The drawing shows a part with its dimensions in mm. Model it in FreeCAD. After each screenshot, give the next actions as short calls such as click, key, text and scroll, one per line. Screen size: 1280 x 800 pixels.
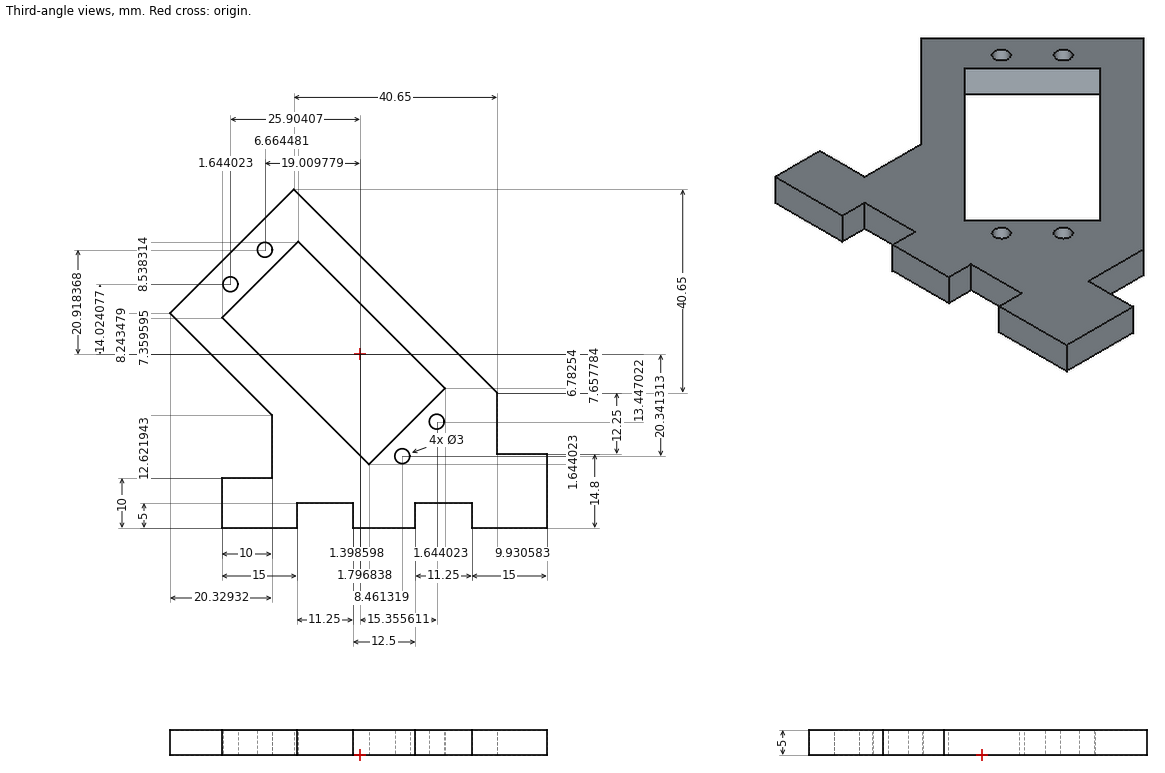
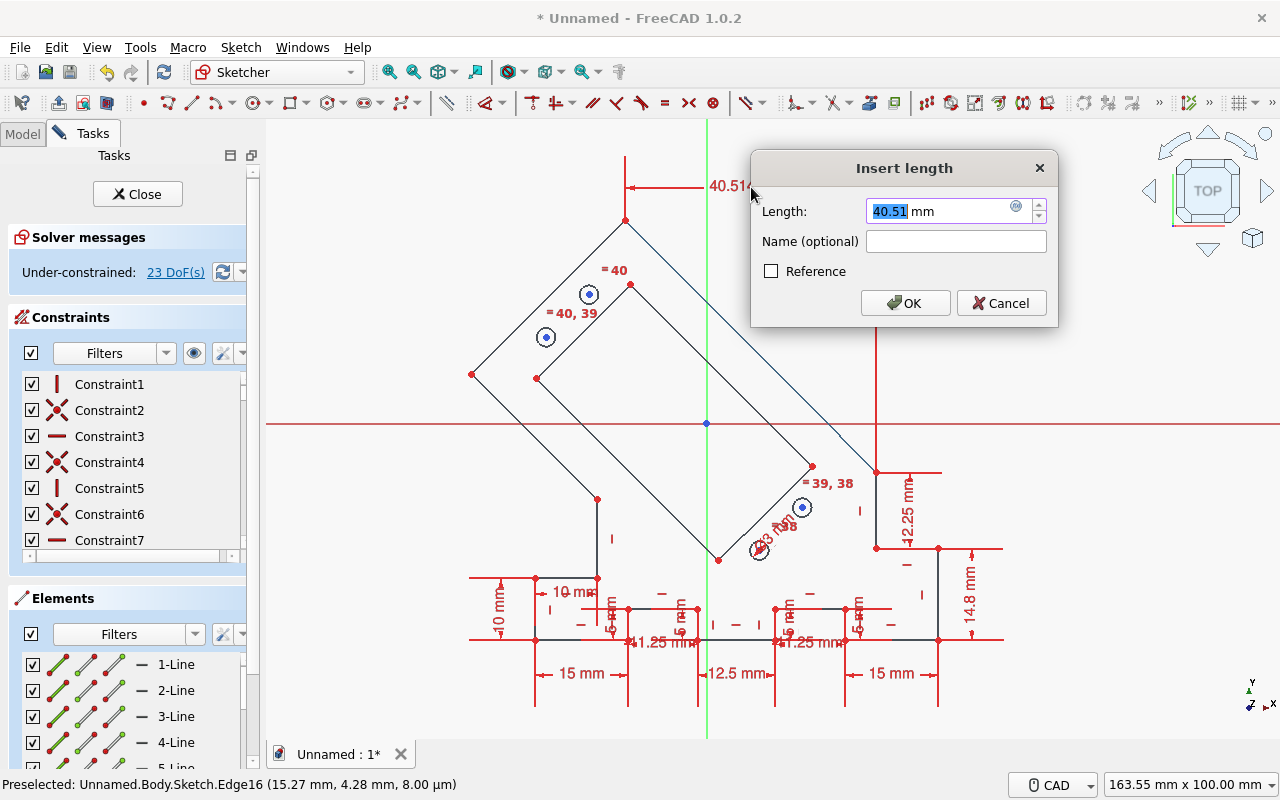
text(40.65)
key(Return)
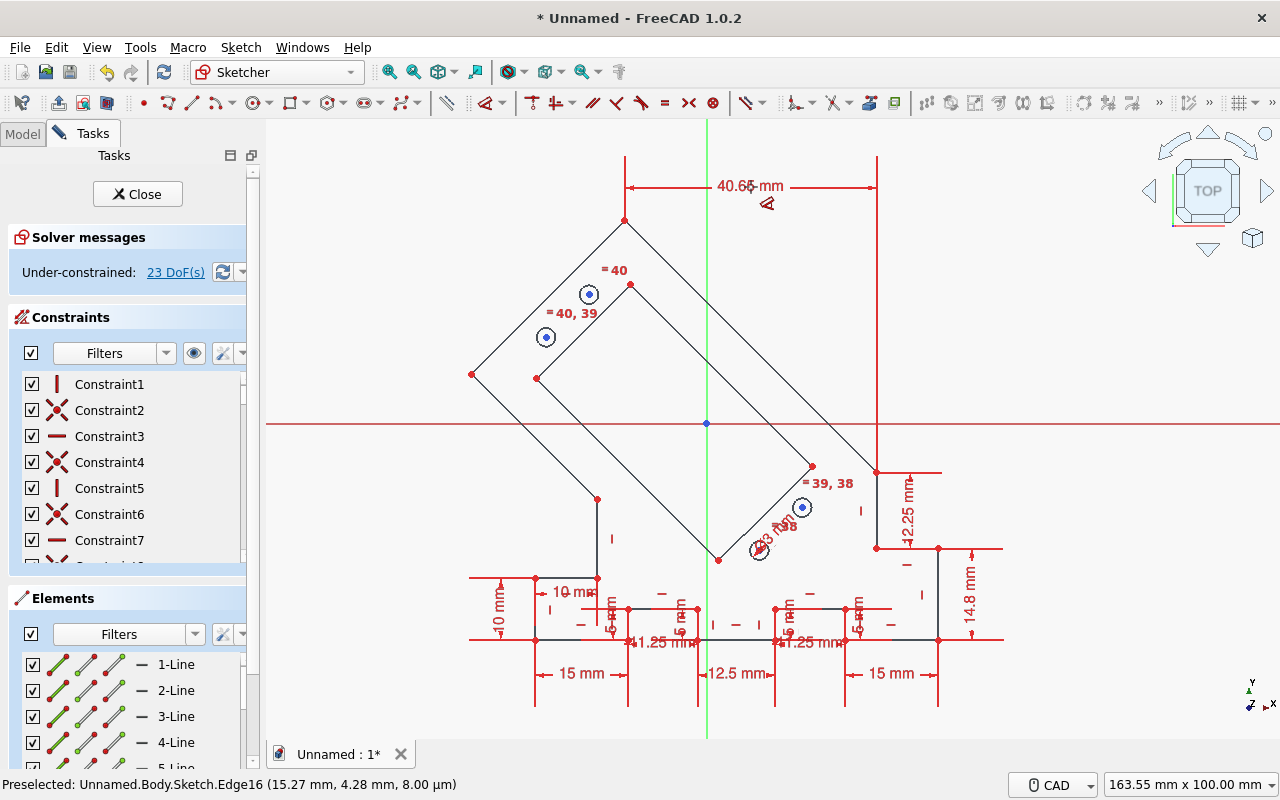
click(801, 397)
click(911, 347)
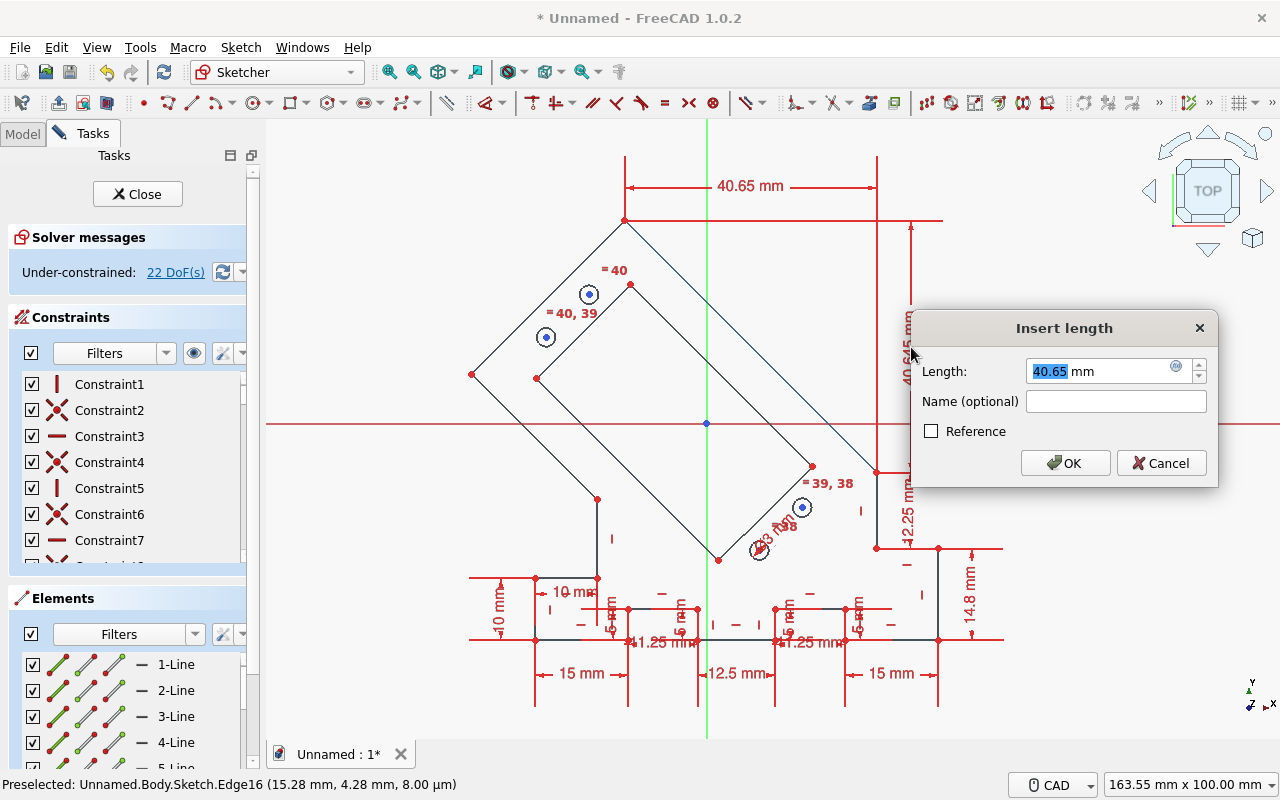
text(40.65)
key(Return)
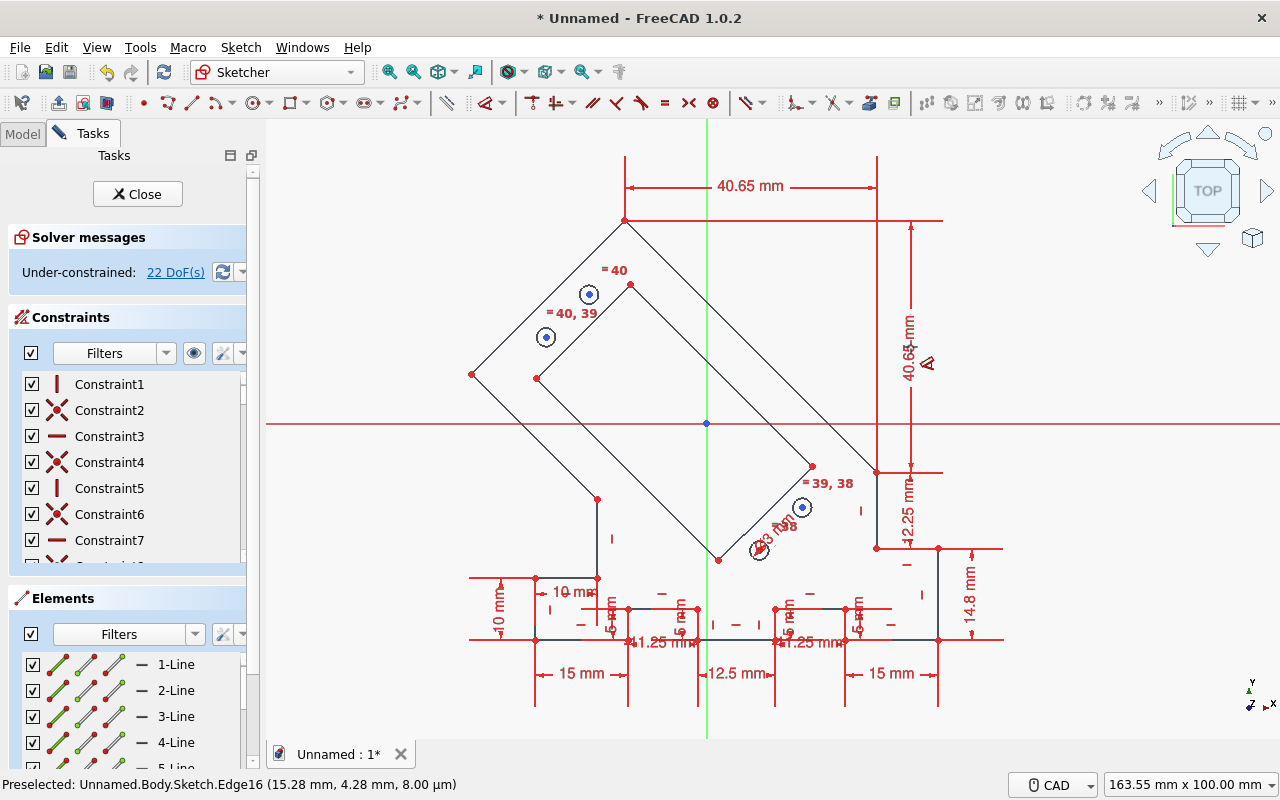
click(920, 549)
click(893, 583)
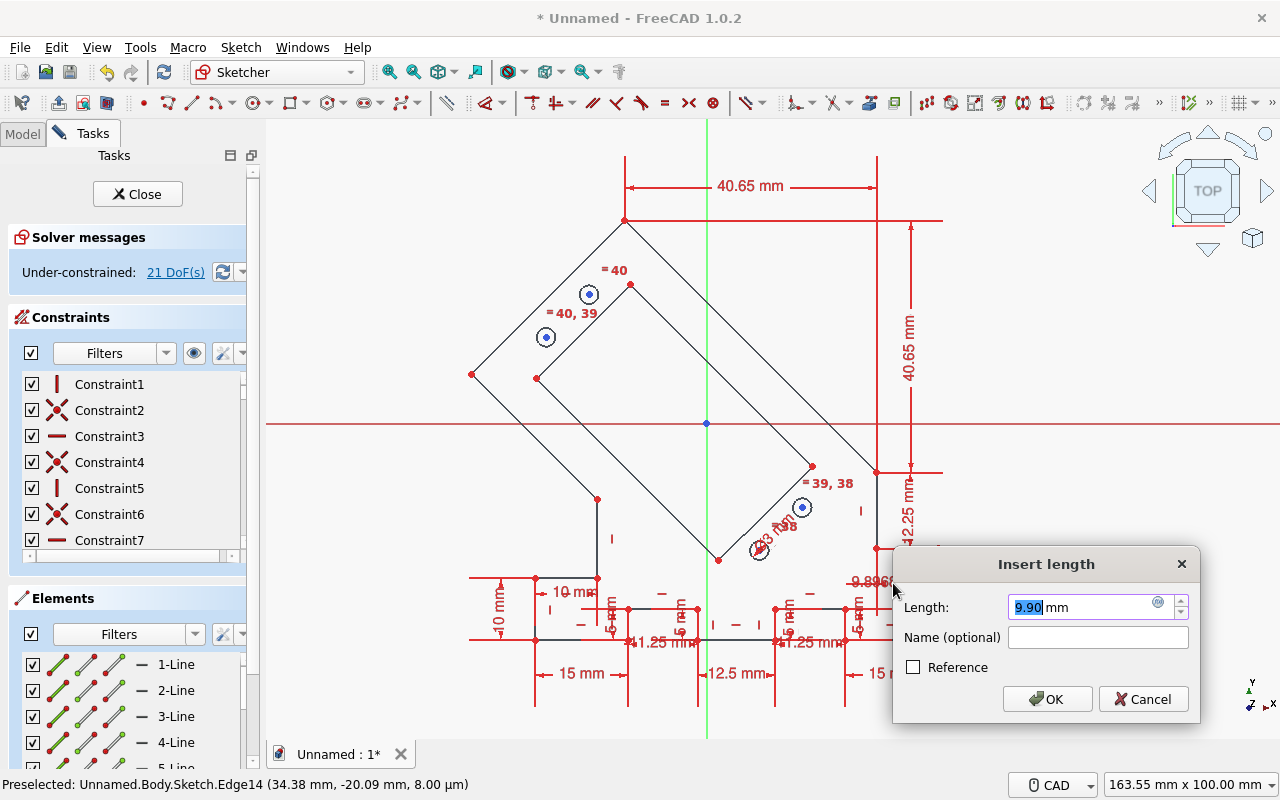
text(9.930583)
key(Return)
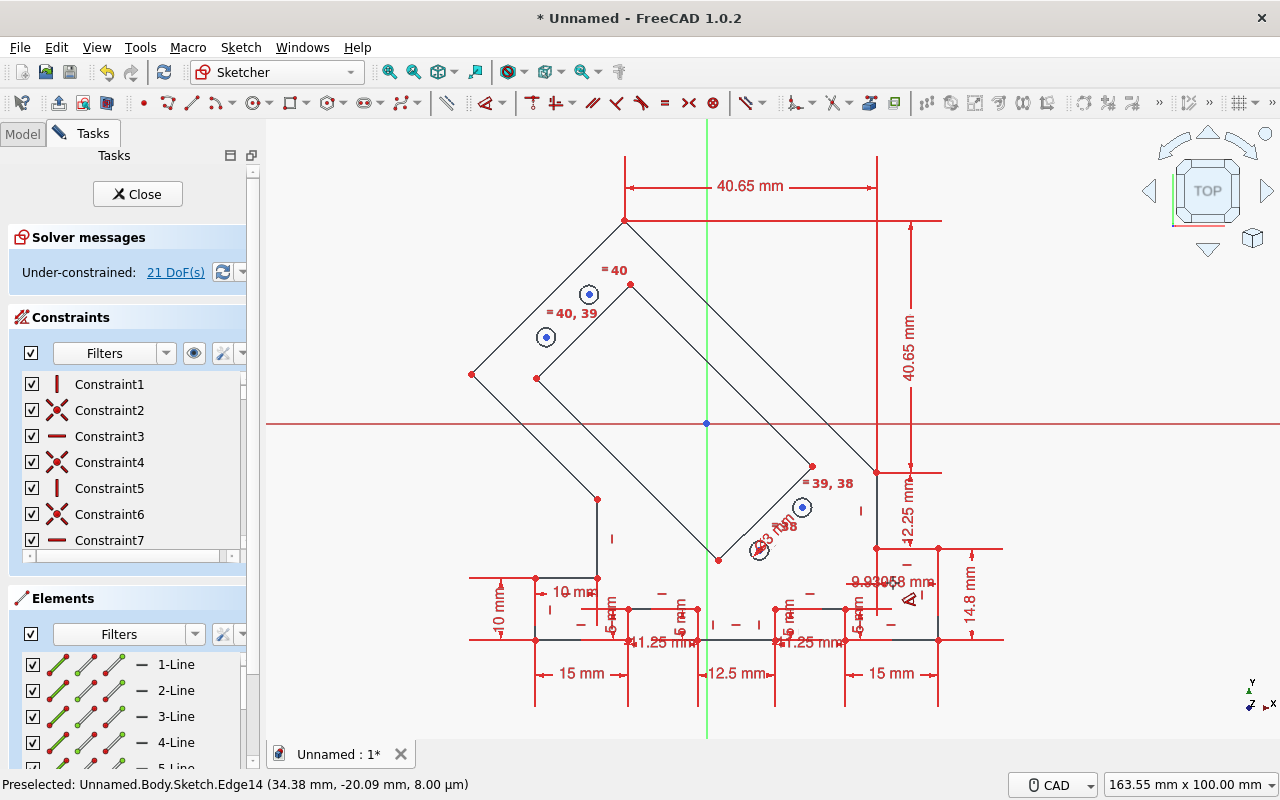
click(813, 467)
click(673, 445)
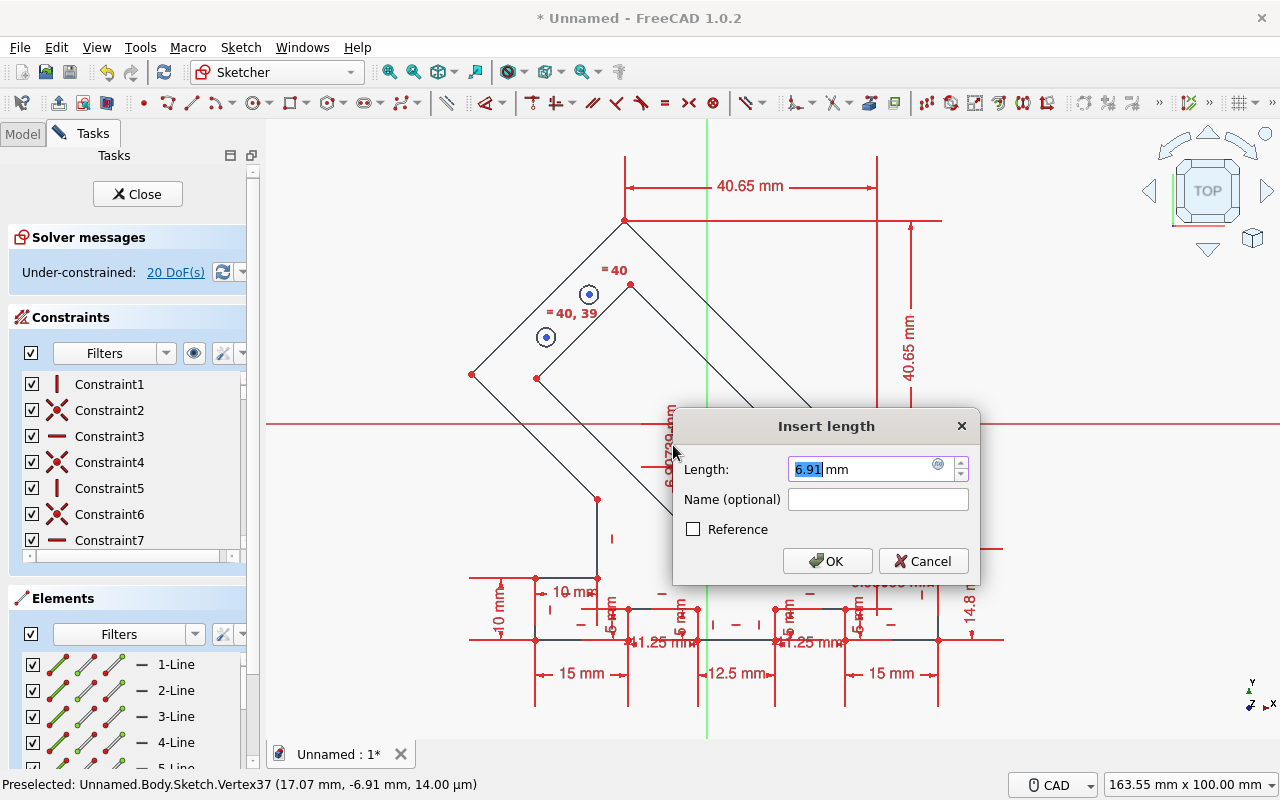
text(6.78254)
key(Return)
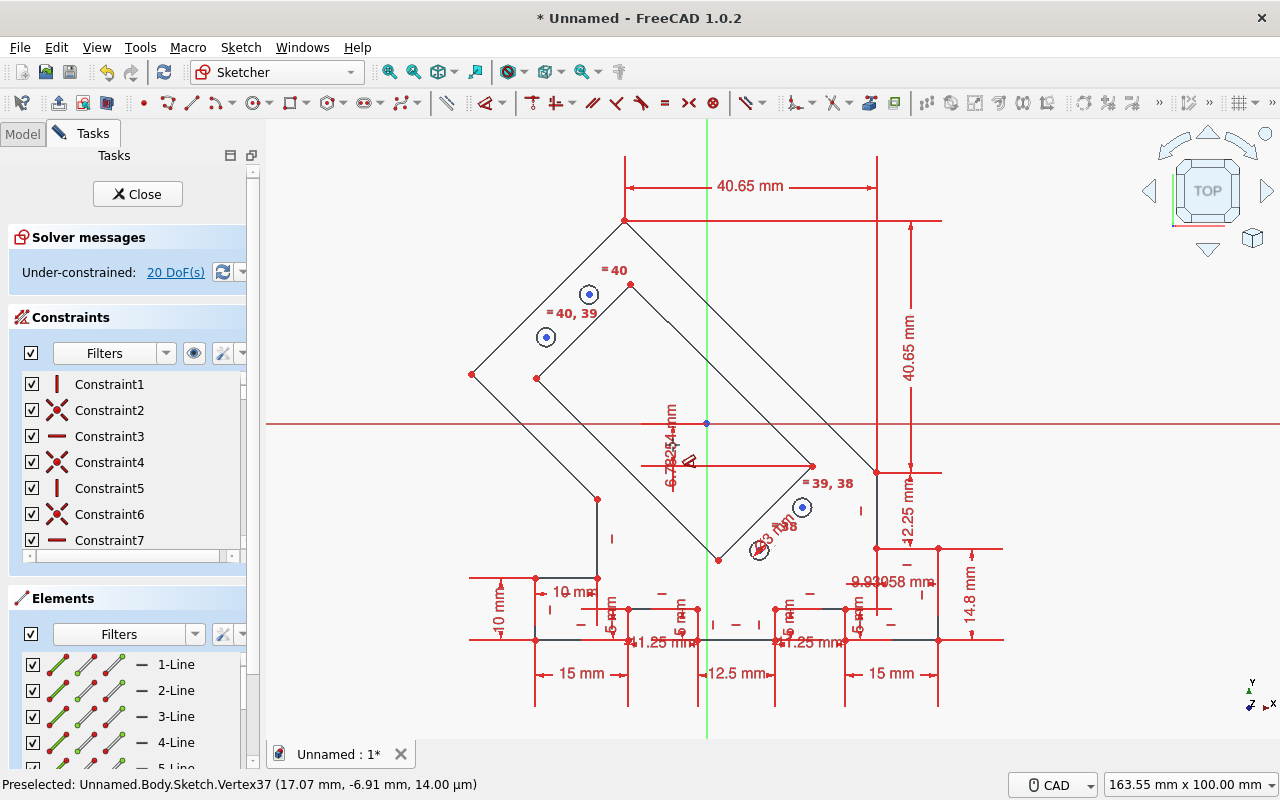
click(759, 551)
click(733, 585)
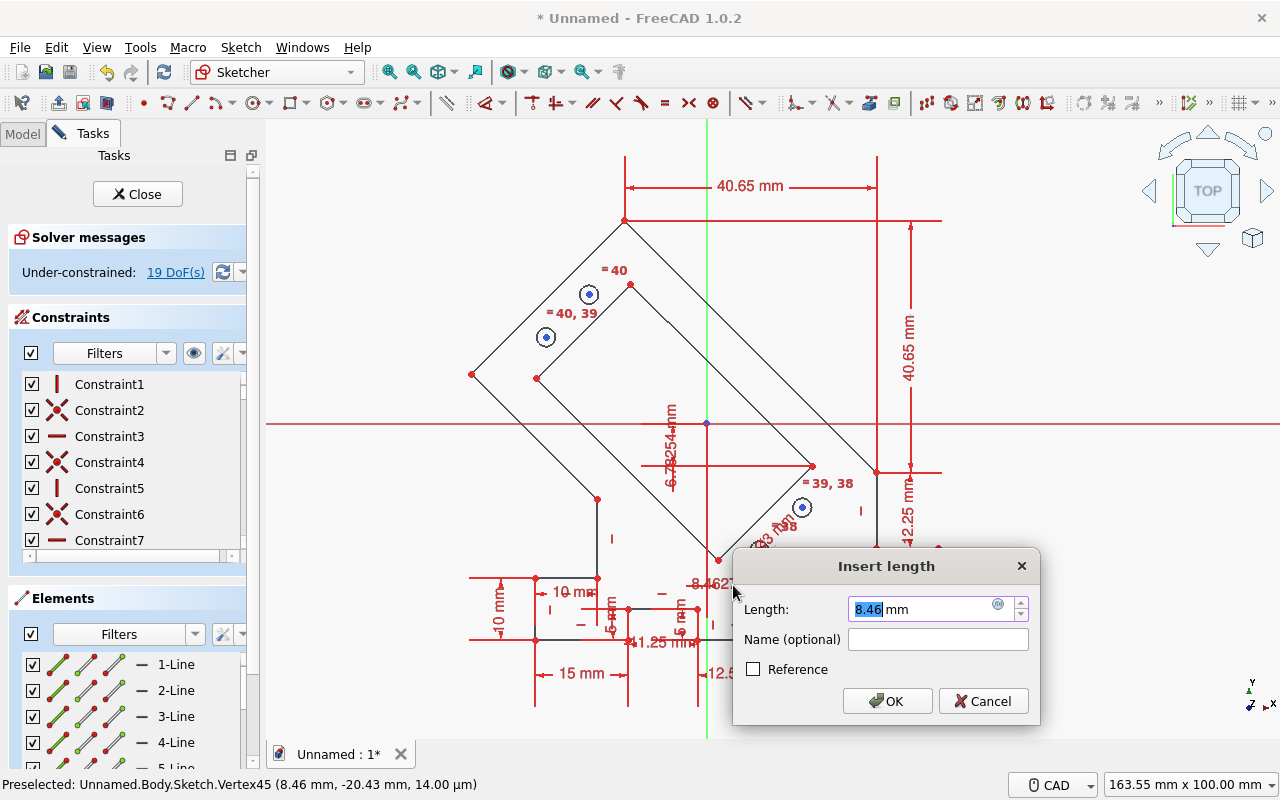
text(8.461319)
key(Return)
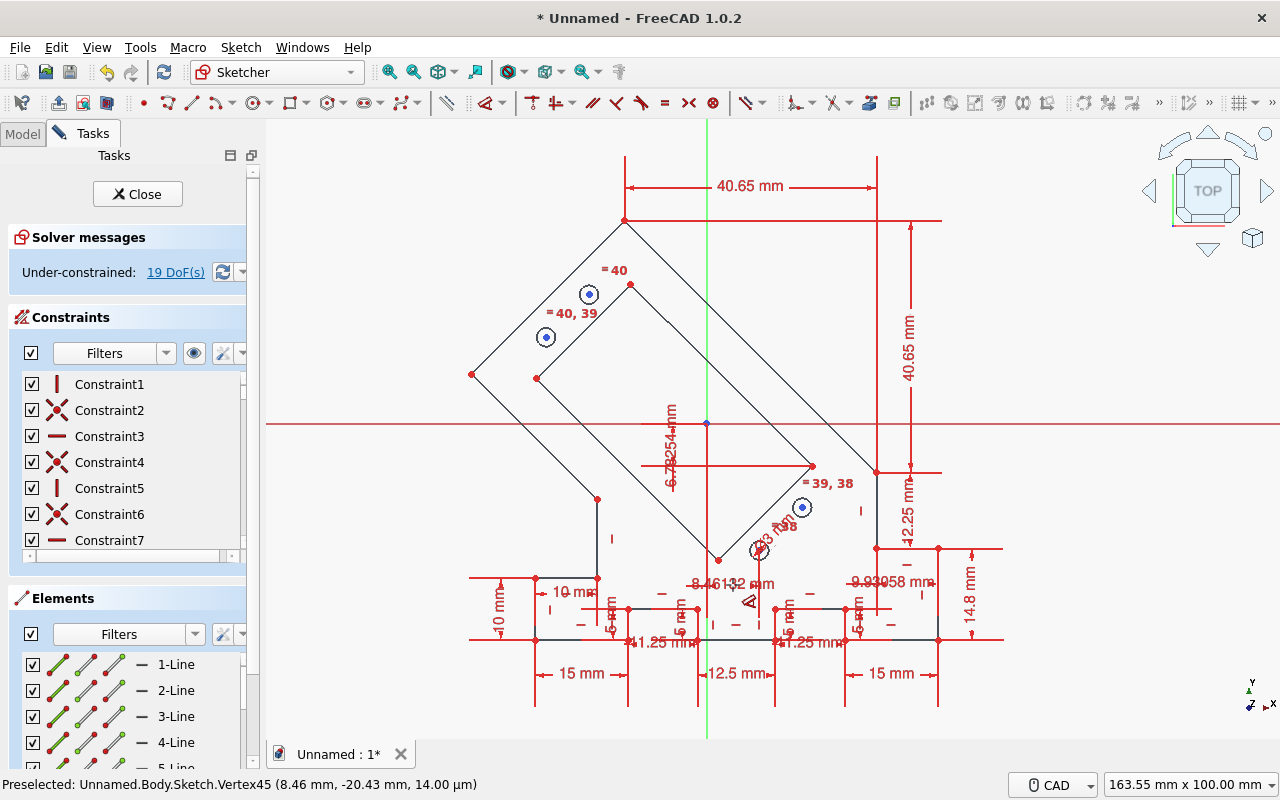
click(546, 337)
click(683, 303)